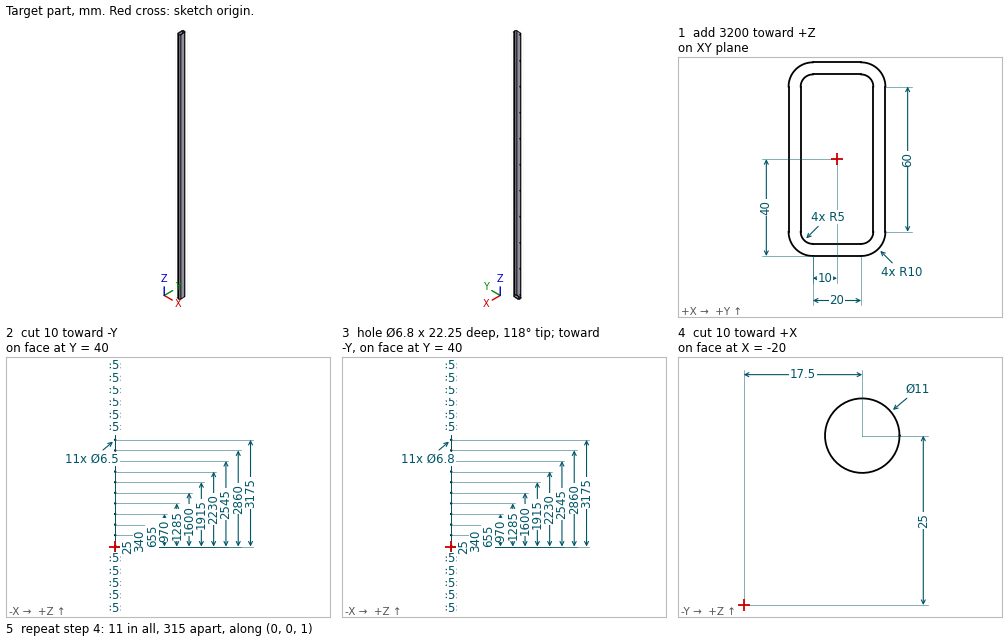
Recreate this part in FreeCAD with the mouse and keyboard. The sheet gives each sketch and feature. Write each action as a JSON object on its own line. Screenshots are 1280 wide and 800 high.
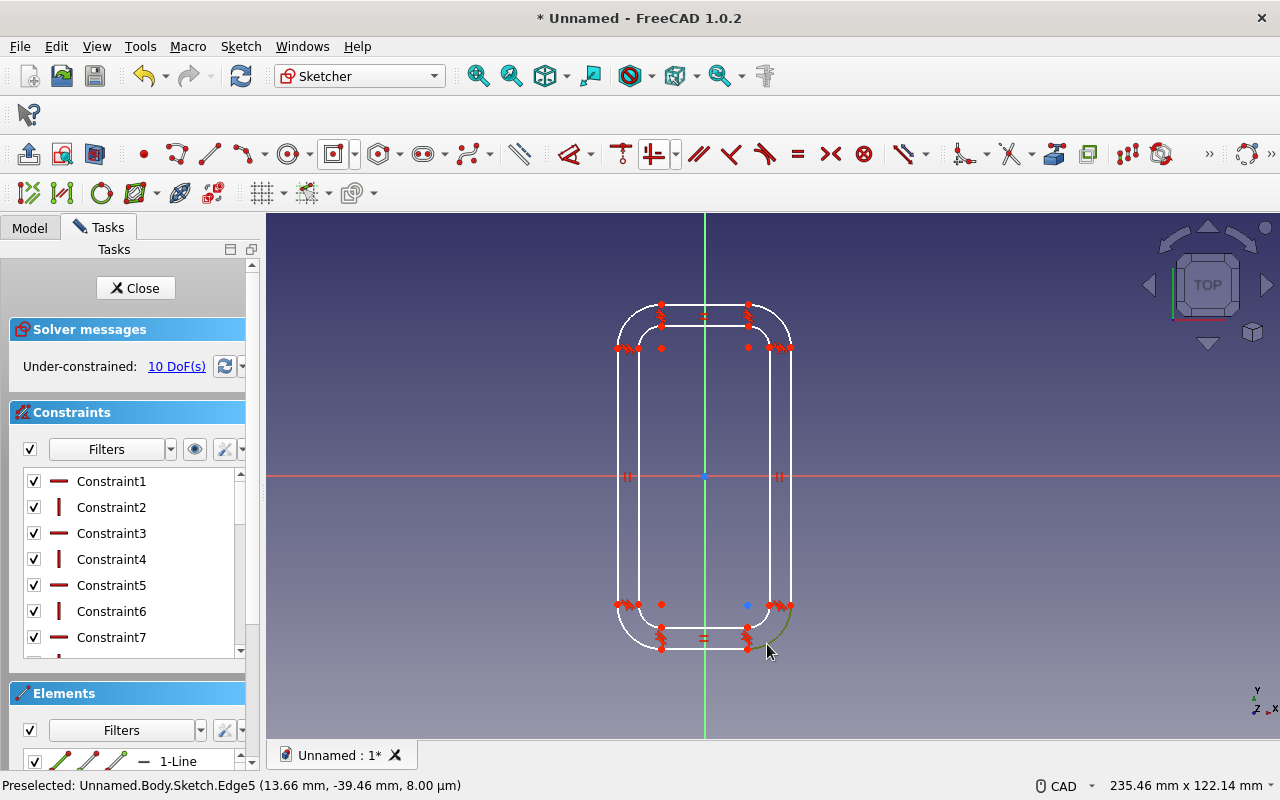
{"action": "left_click", "coordinate": [786, 328]}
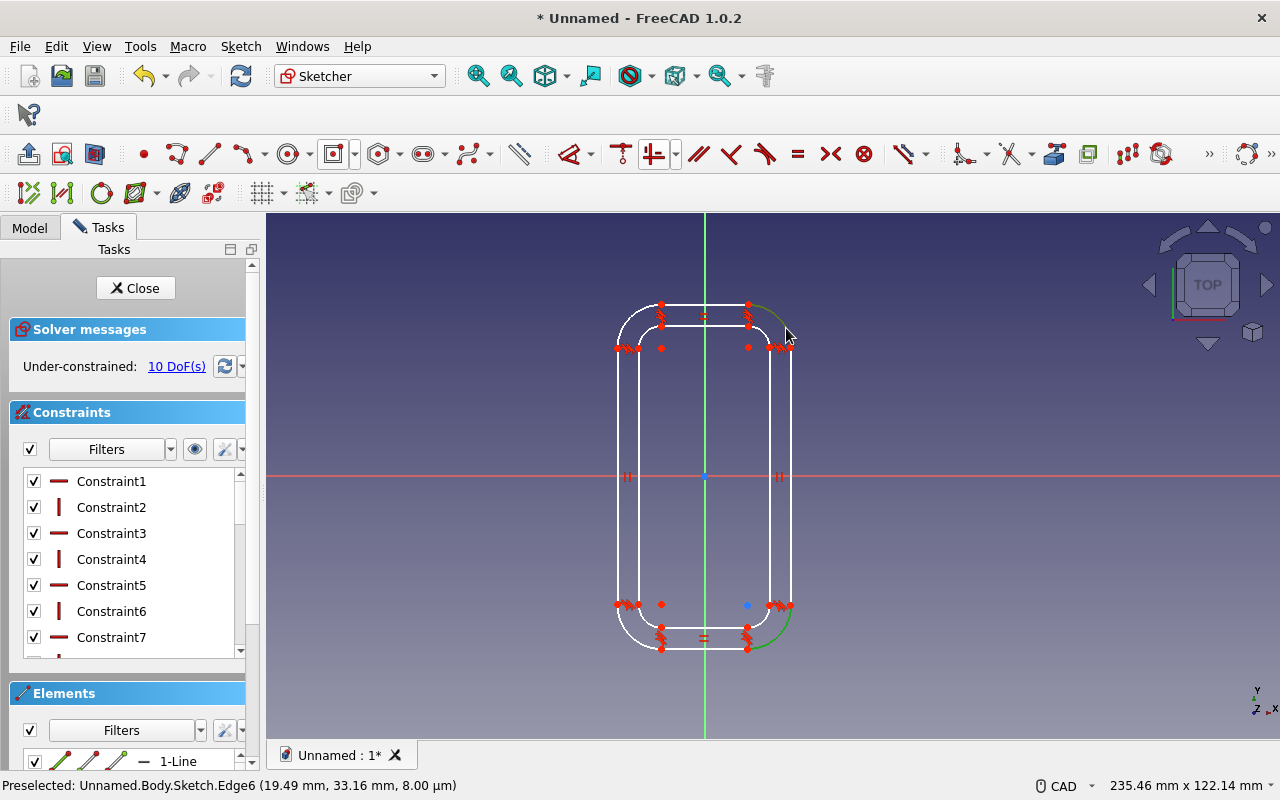
{"action": "left_click", "coordinate": [641, 310]}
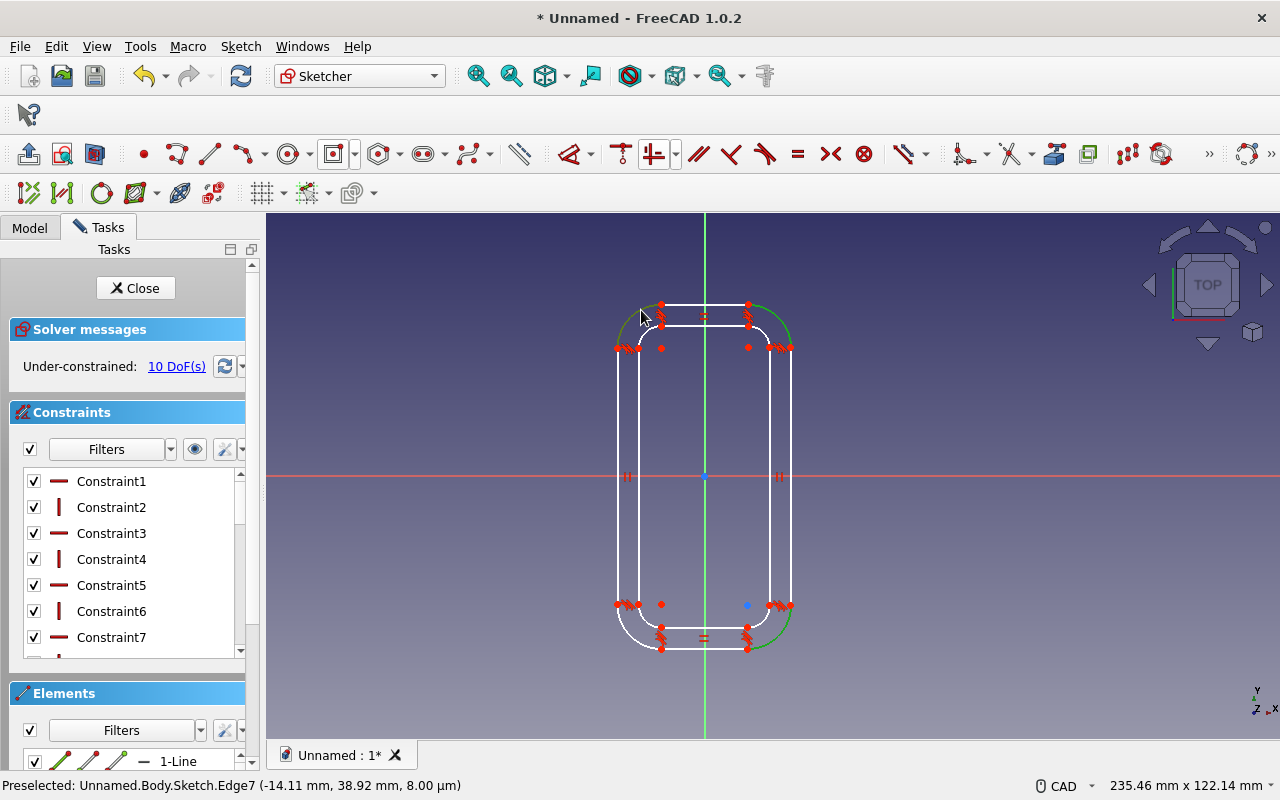
{"action": "left_click", "coordinate": [622, 625]}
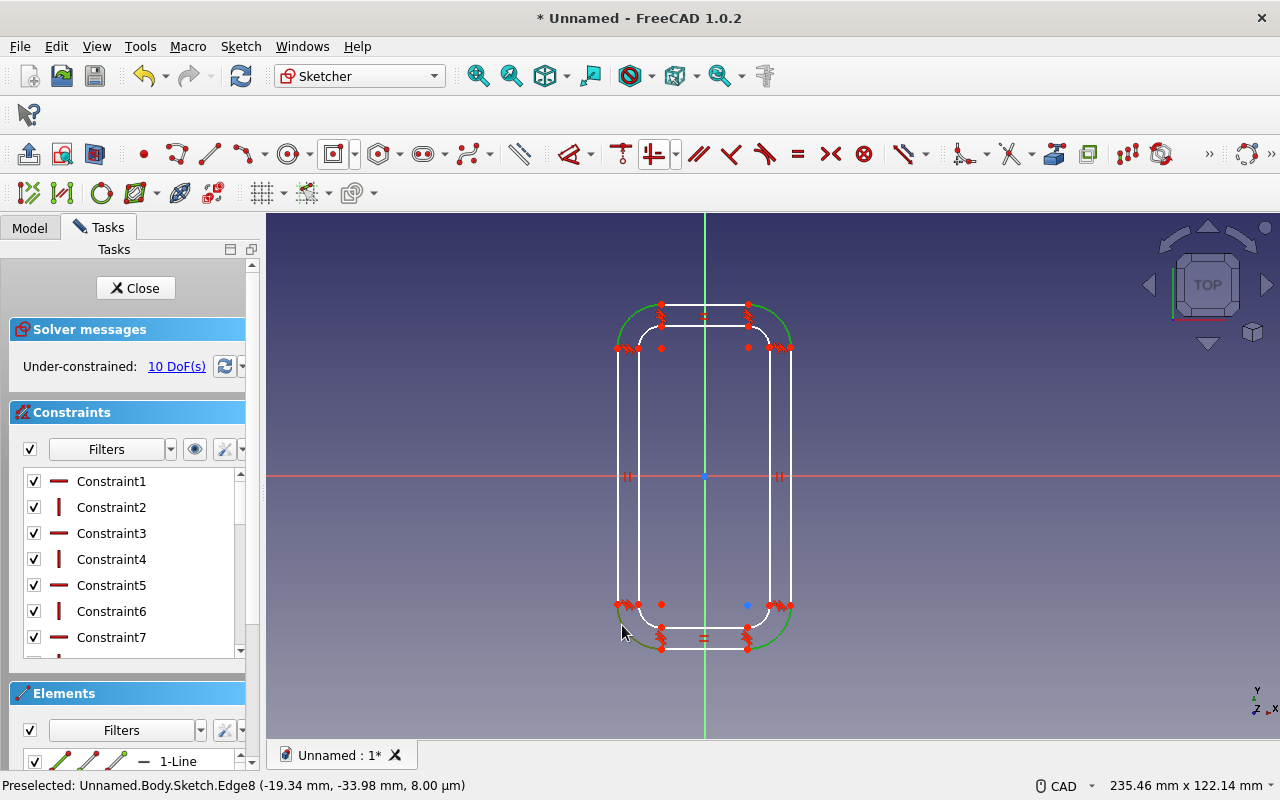
{"action": "left_click", "coordinate": [798, 154]}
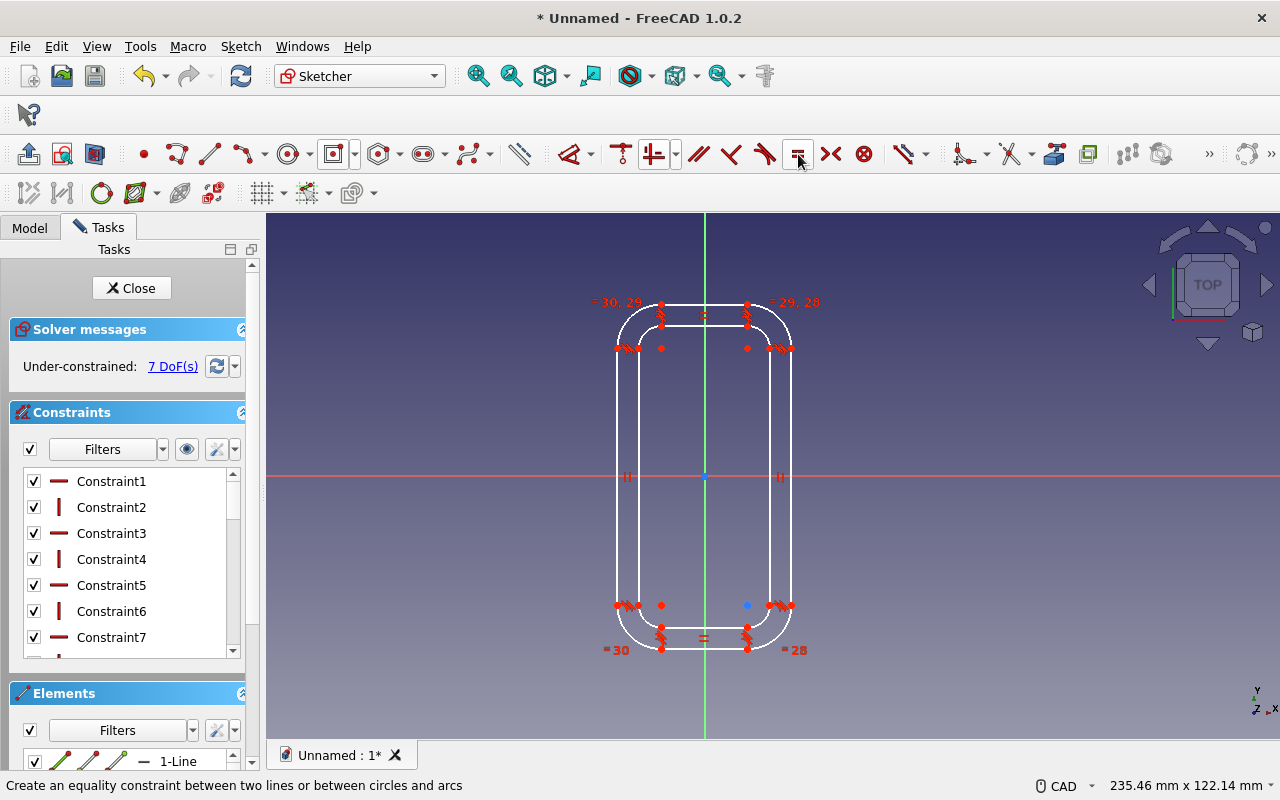
{"action": "scroll", "coordinate": [641, 615], "scroll_direction": "up", "scroll_amount": 2}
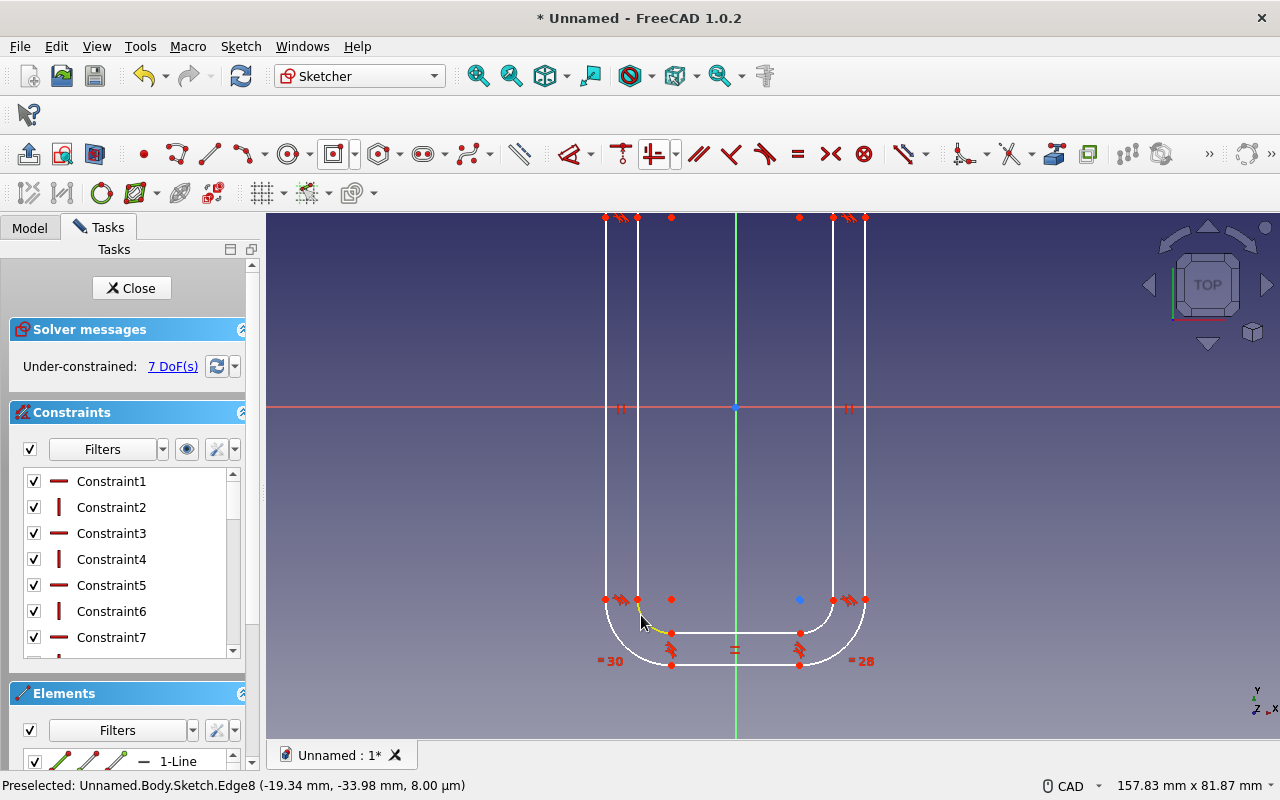
{"action": "left_click", "coordinate": [641, 615]}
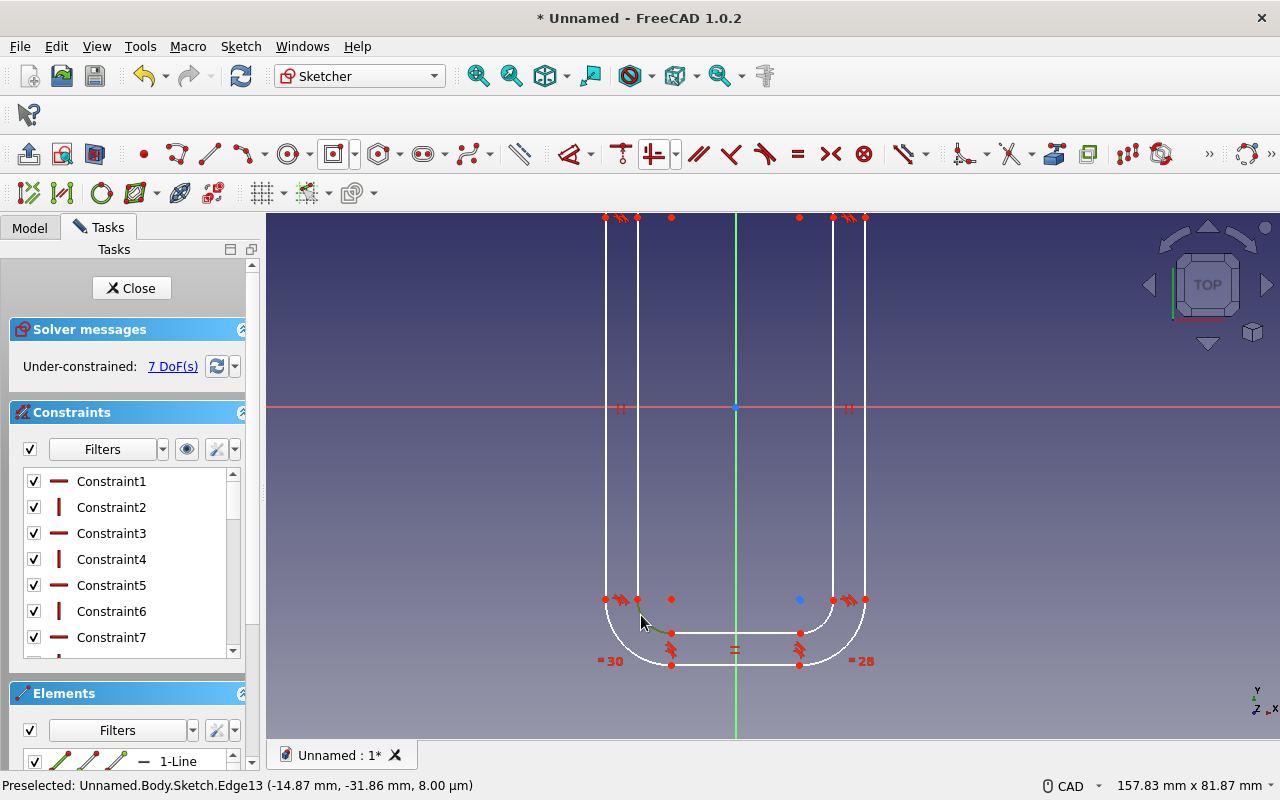
{"action": "left_click", "coordinate": [815, 630]}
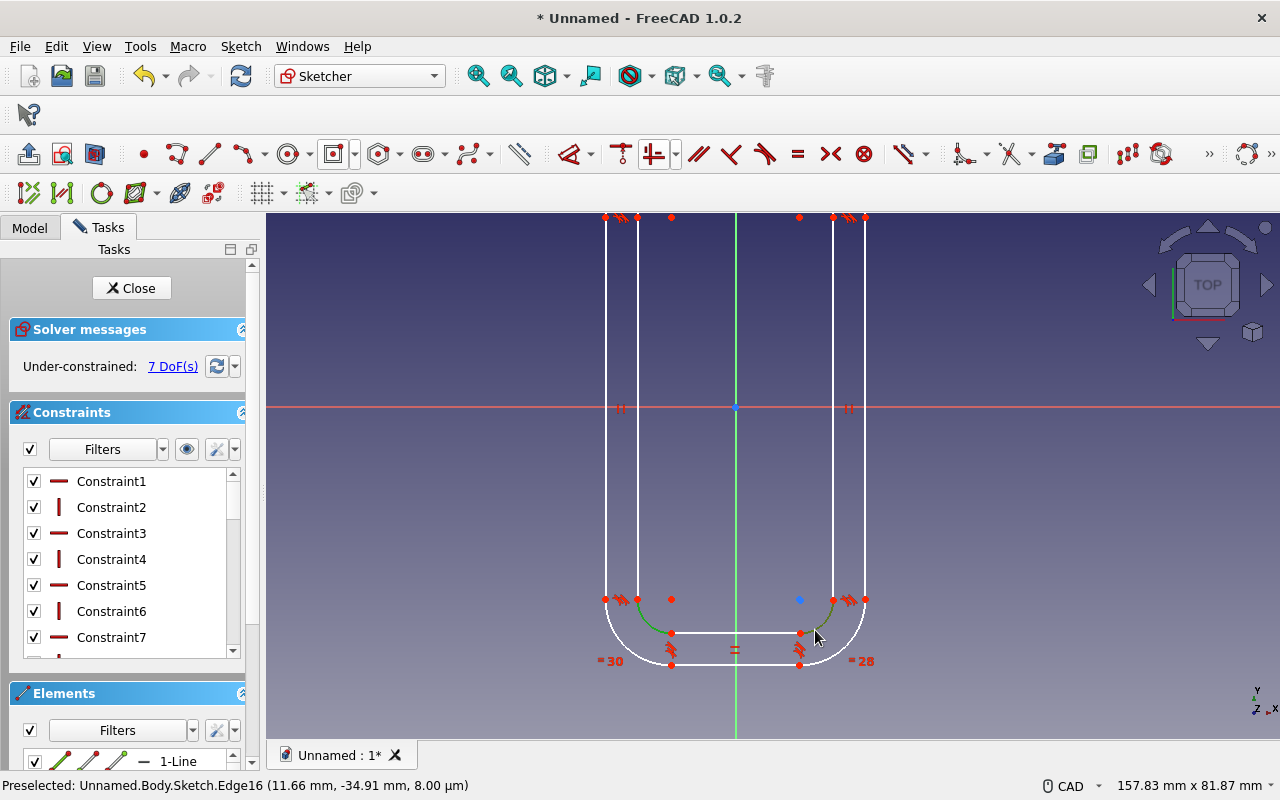
{"action": "left_click", "coordinate": [798, 154]}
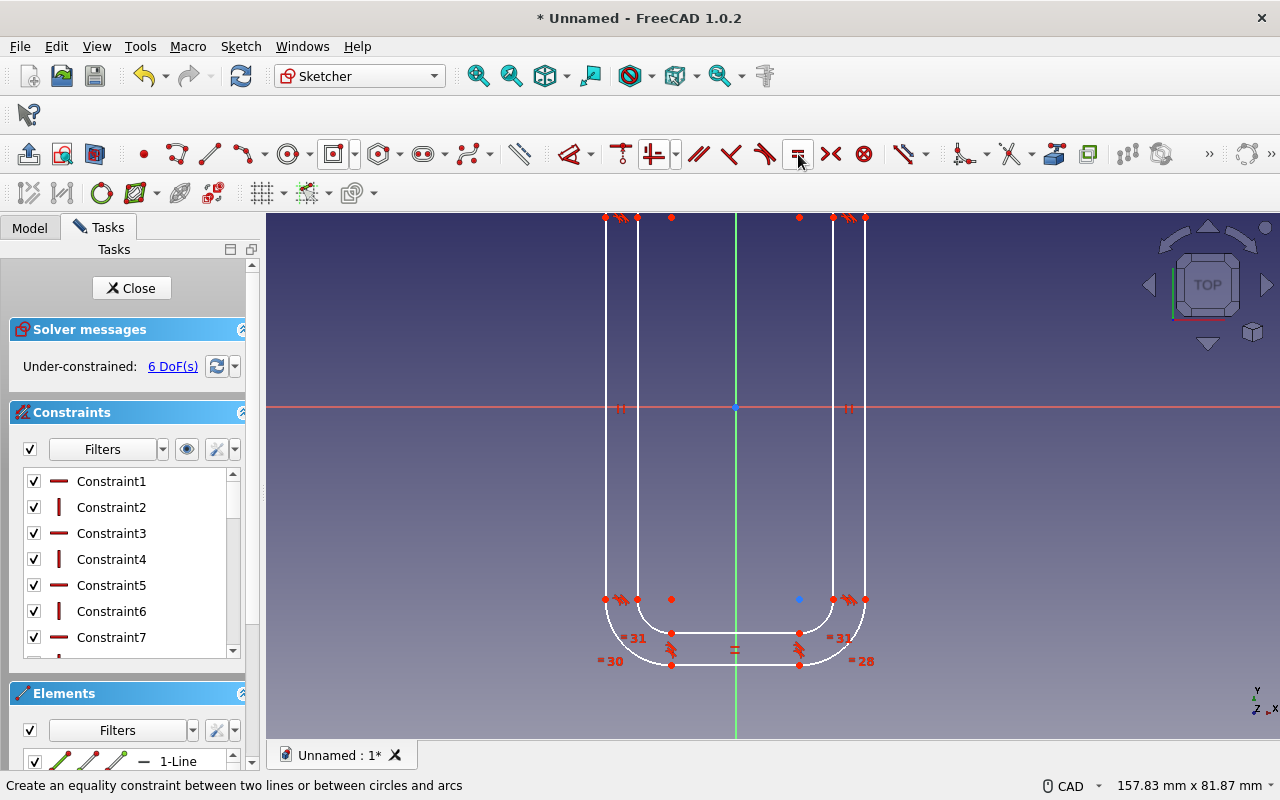
{"action": "left_click", "coordinate": [568, 154]}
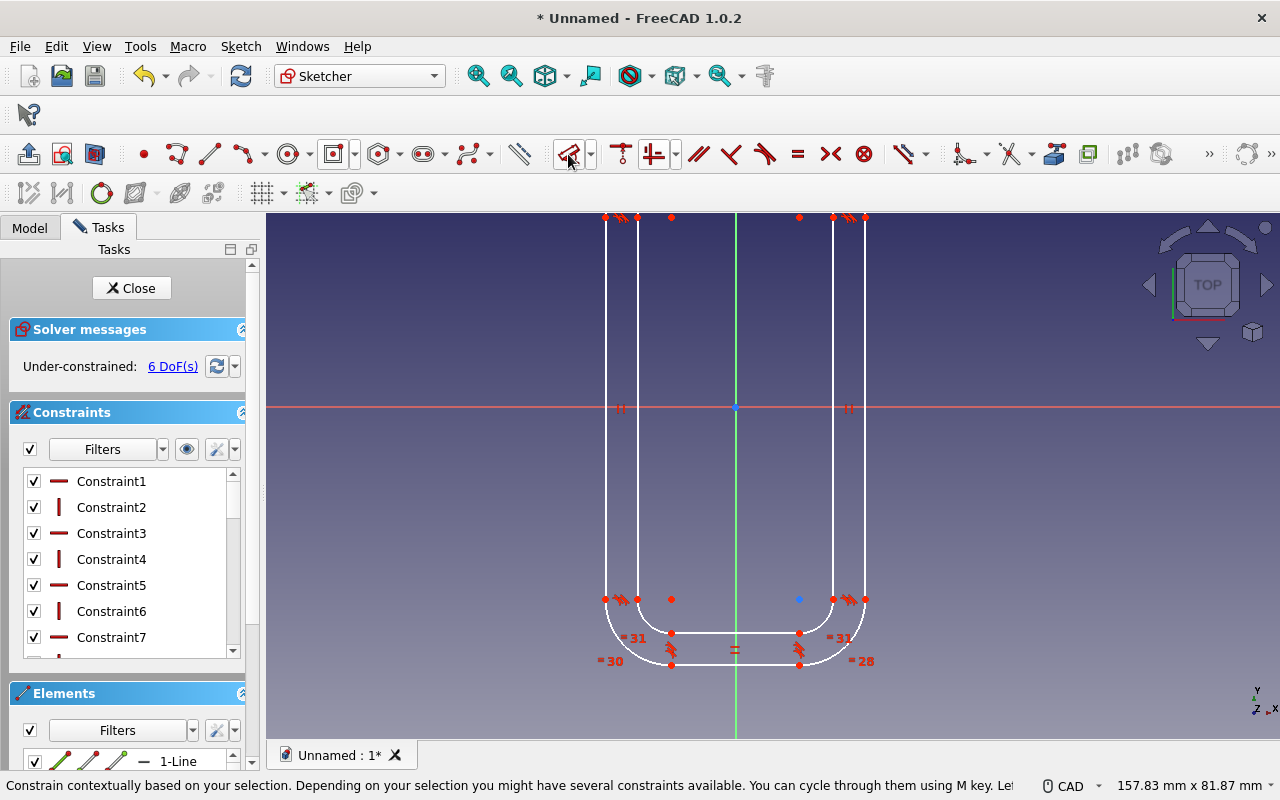
{"action": "left_click", "coordinate": [829, 658]}
{"action": "left_click", "coordinate": [843, 687]}